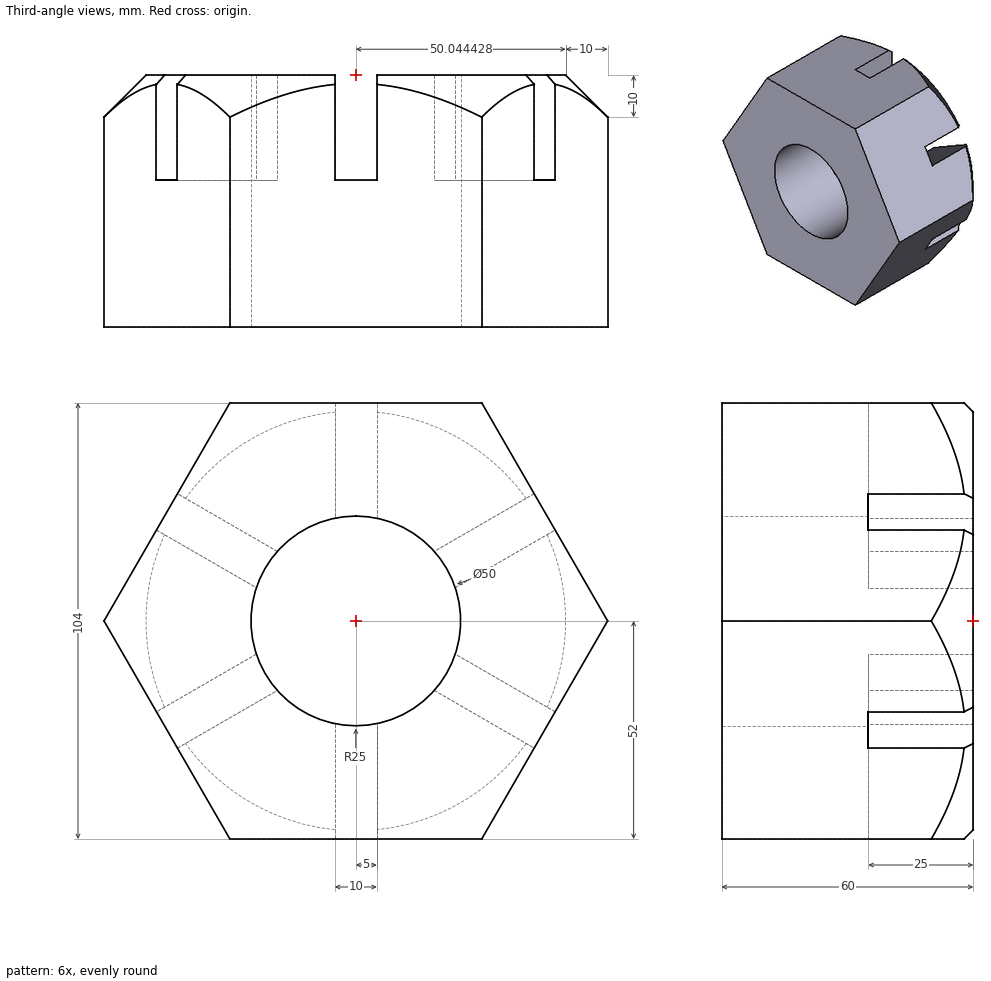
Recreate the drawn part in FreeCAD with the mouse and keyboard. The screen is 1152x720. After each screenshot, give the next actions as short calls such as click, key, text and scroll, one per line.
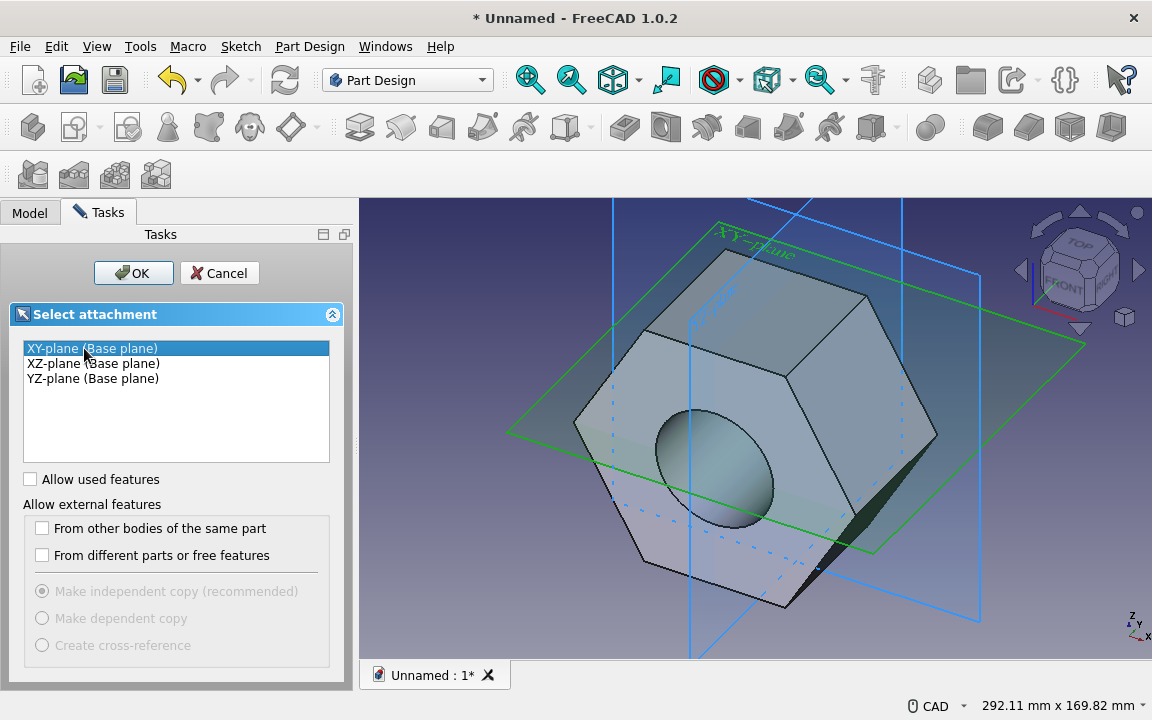
click(134, 273)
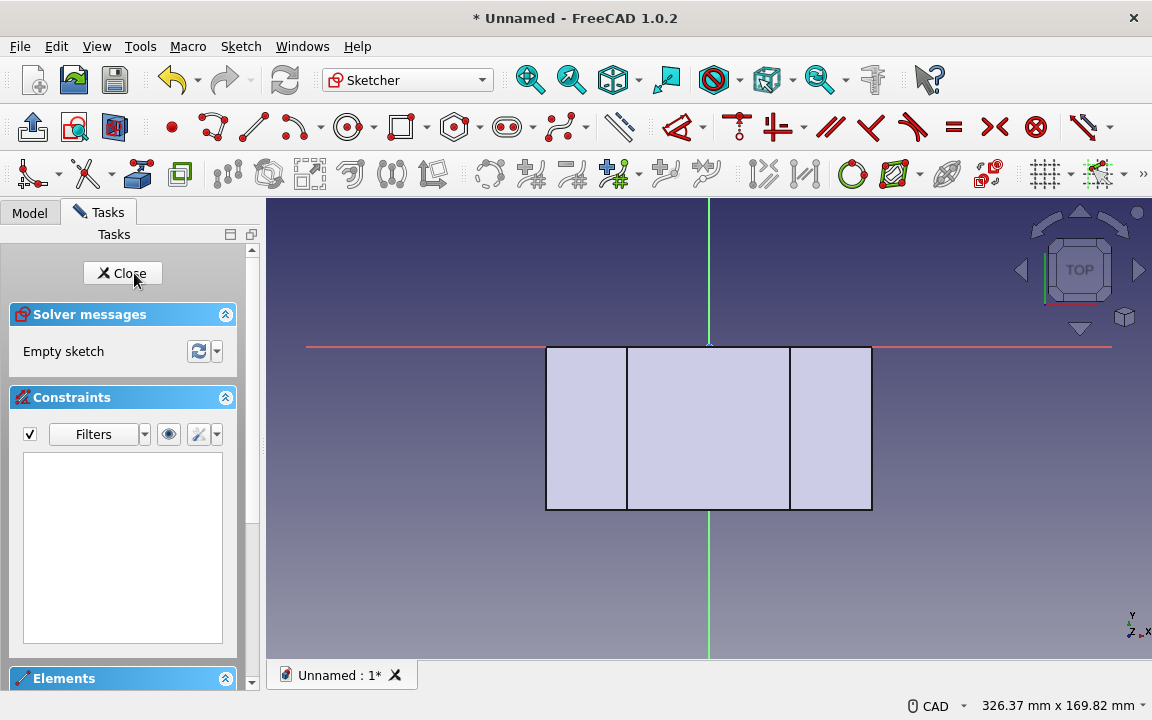
click(115, 128)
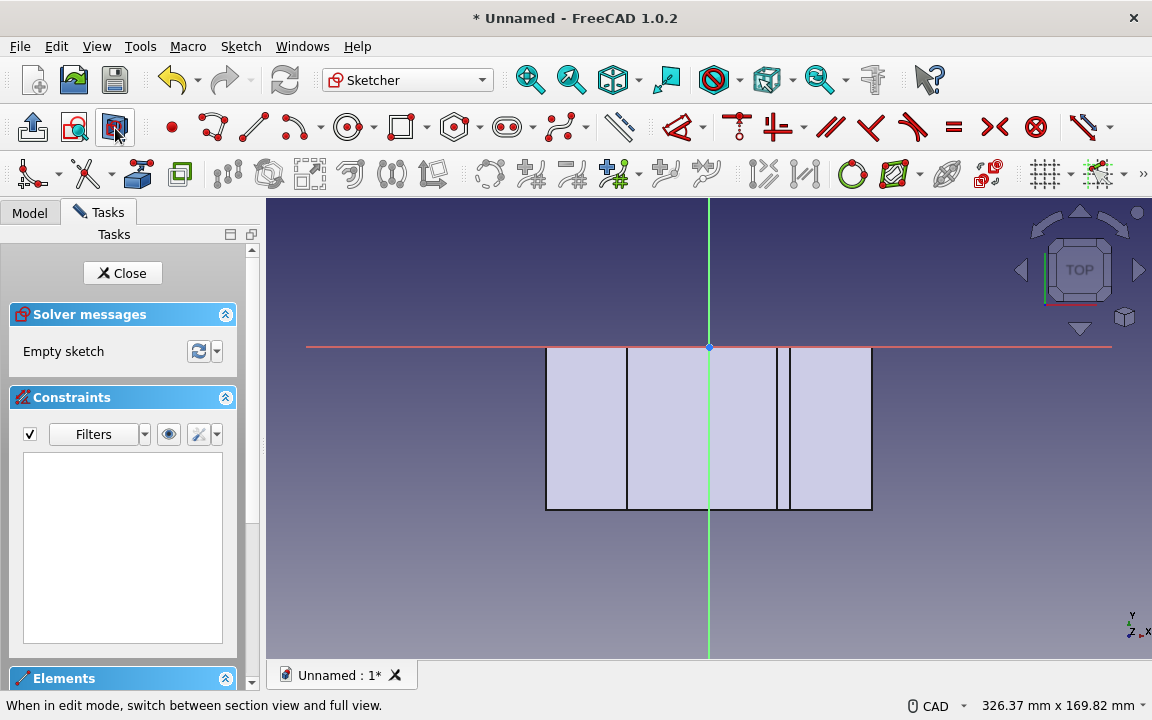
scroll(880, 354, up, 12)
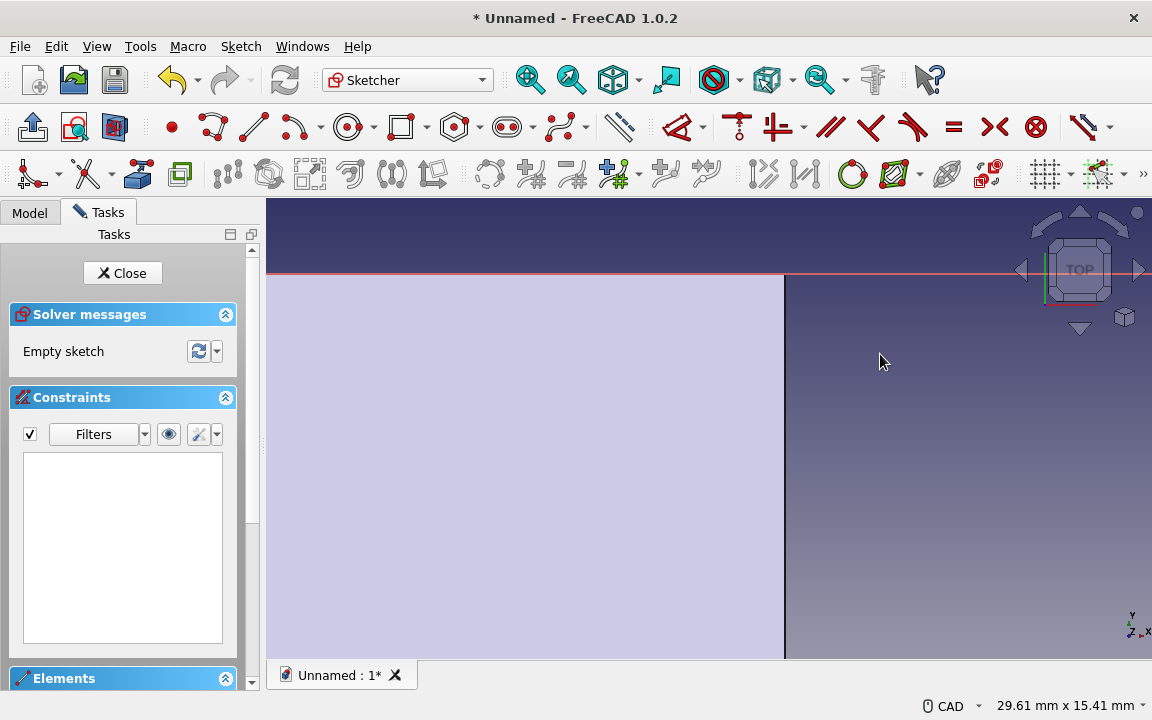
click(213, 128)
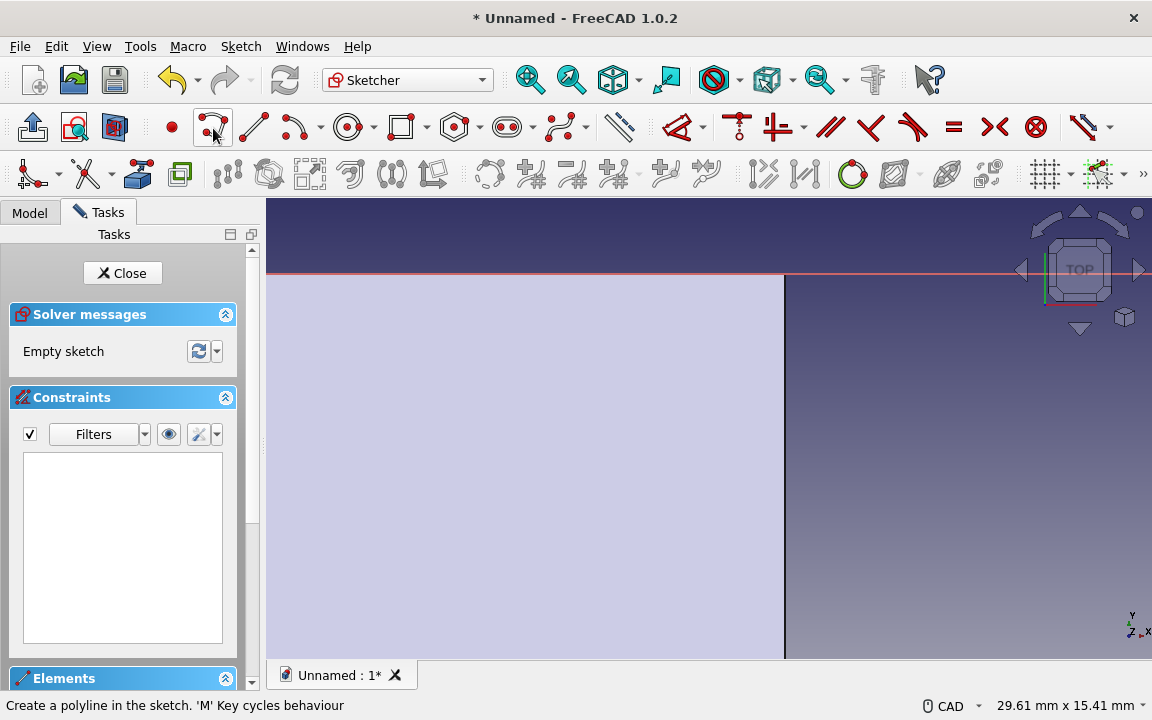
click(486, 274)
click(785, 573)
click(785, 283)
click(486, 274)
key(Escape)
key(Escape)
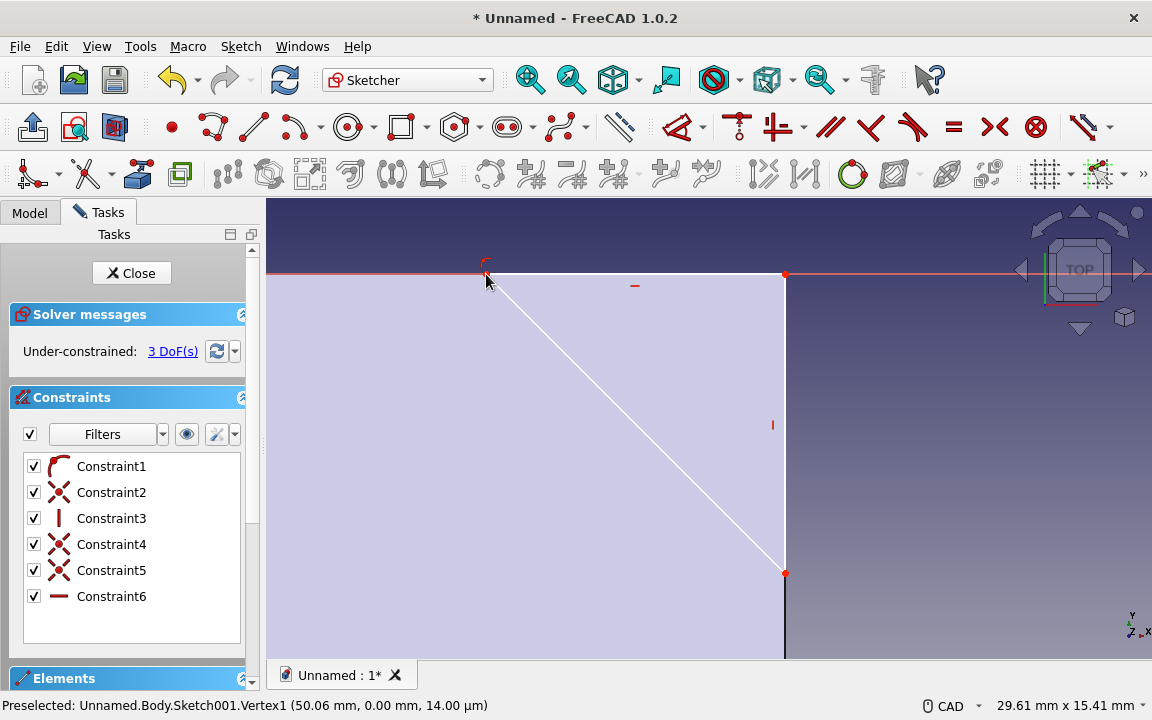
click(676, 128)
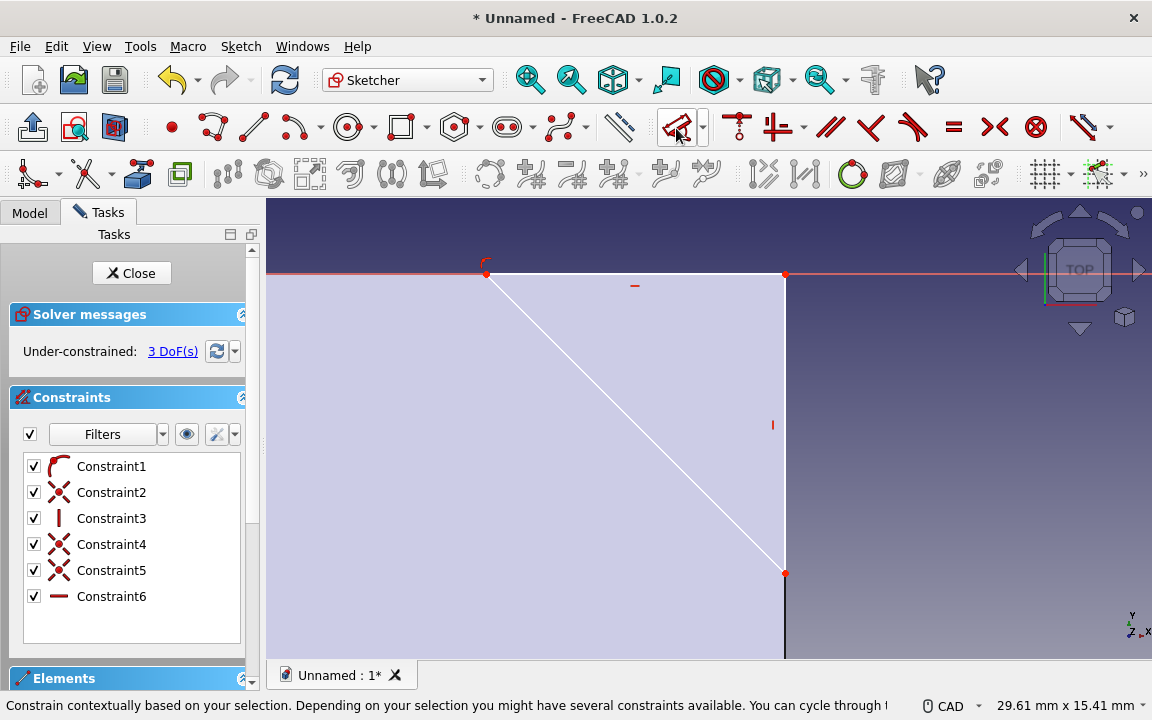
click(785, 484)
click(819, 424)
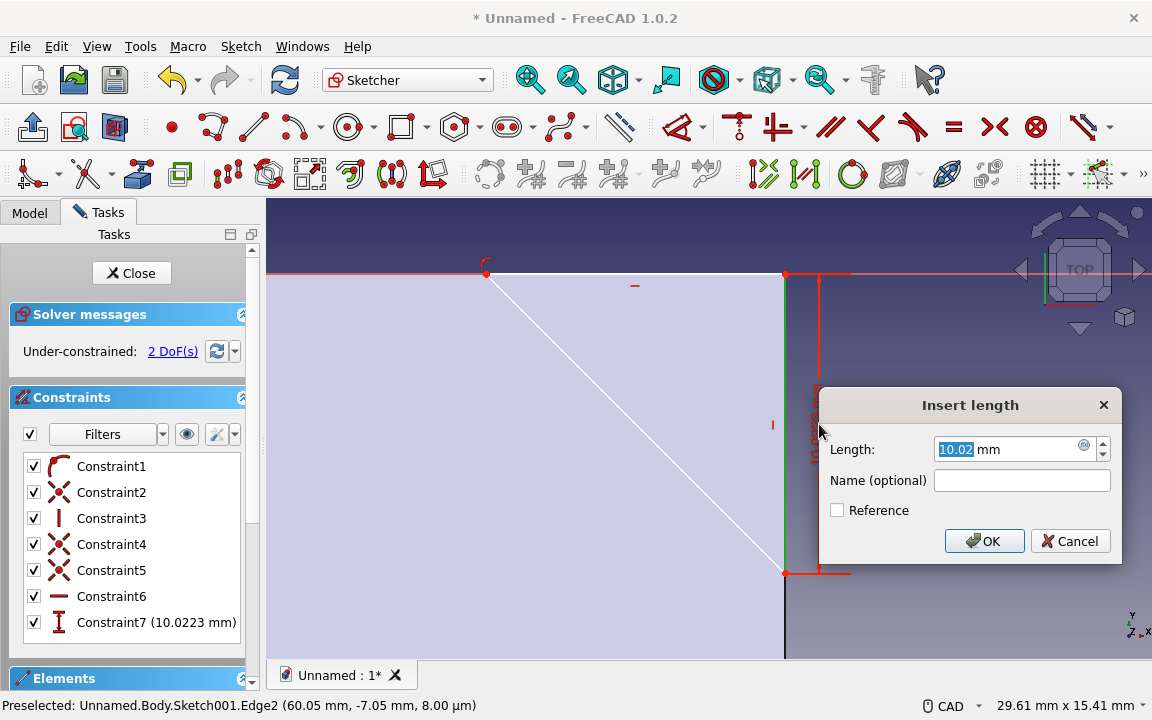
text(10)
key(Return)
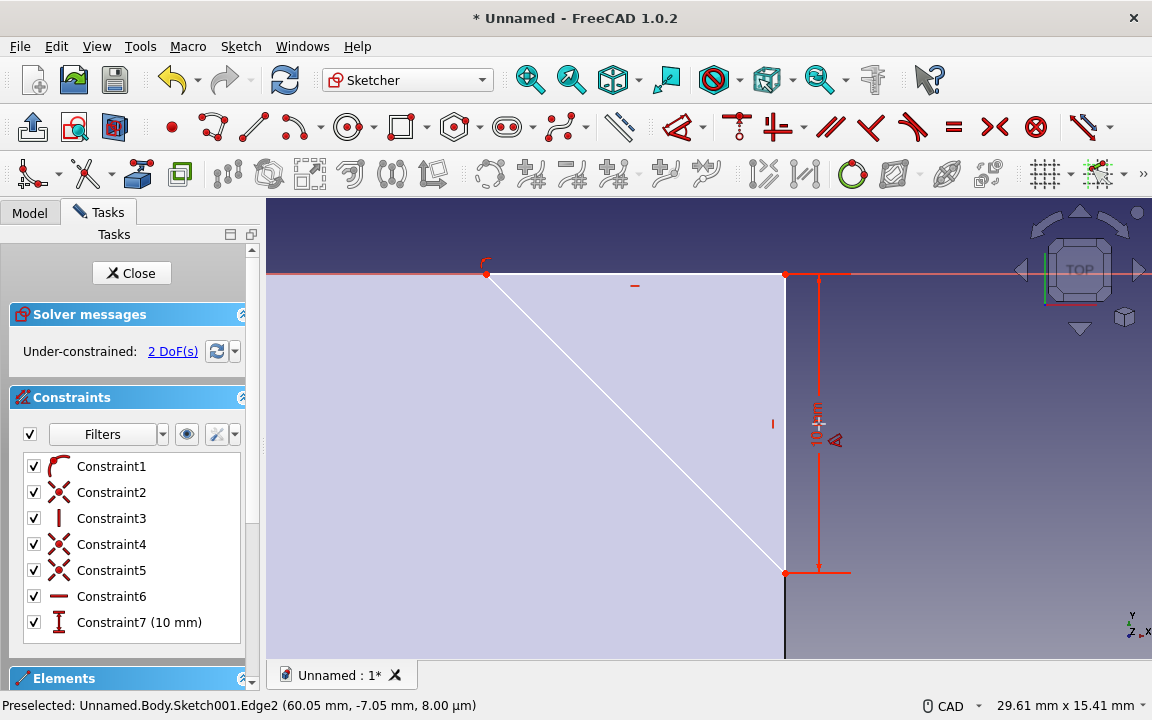
click(695, 274)
click(636, 240)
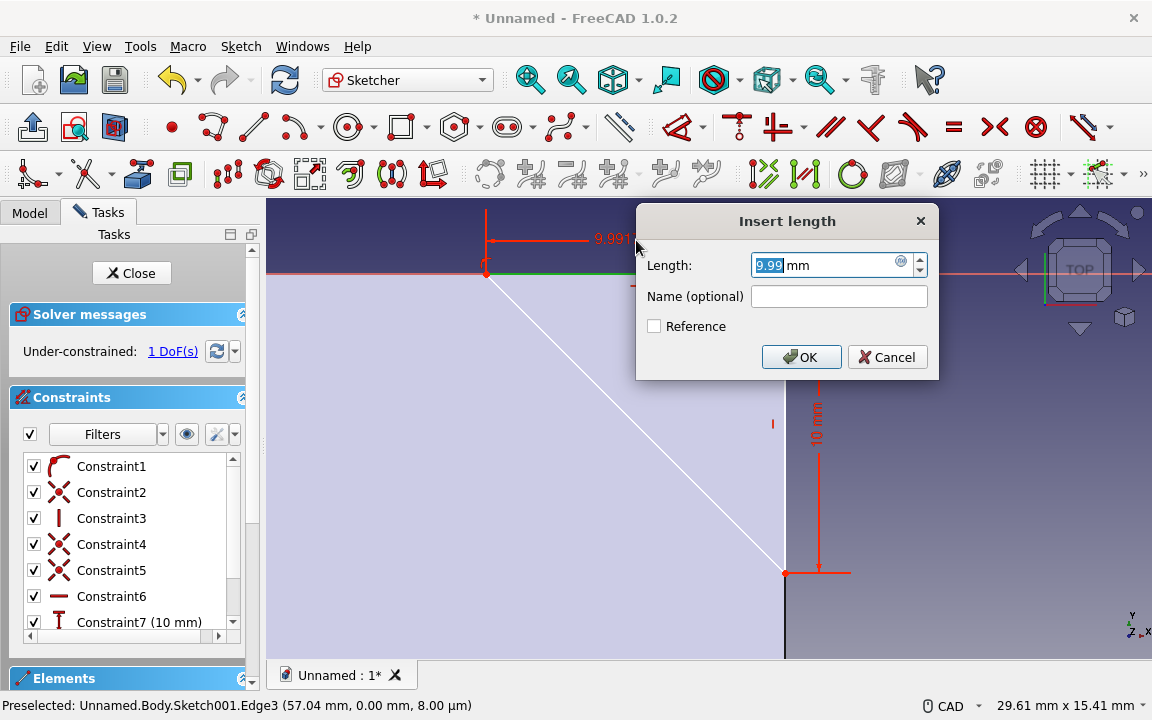
text(10)
key(Return)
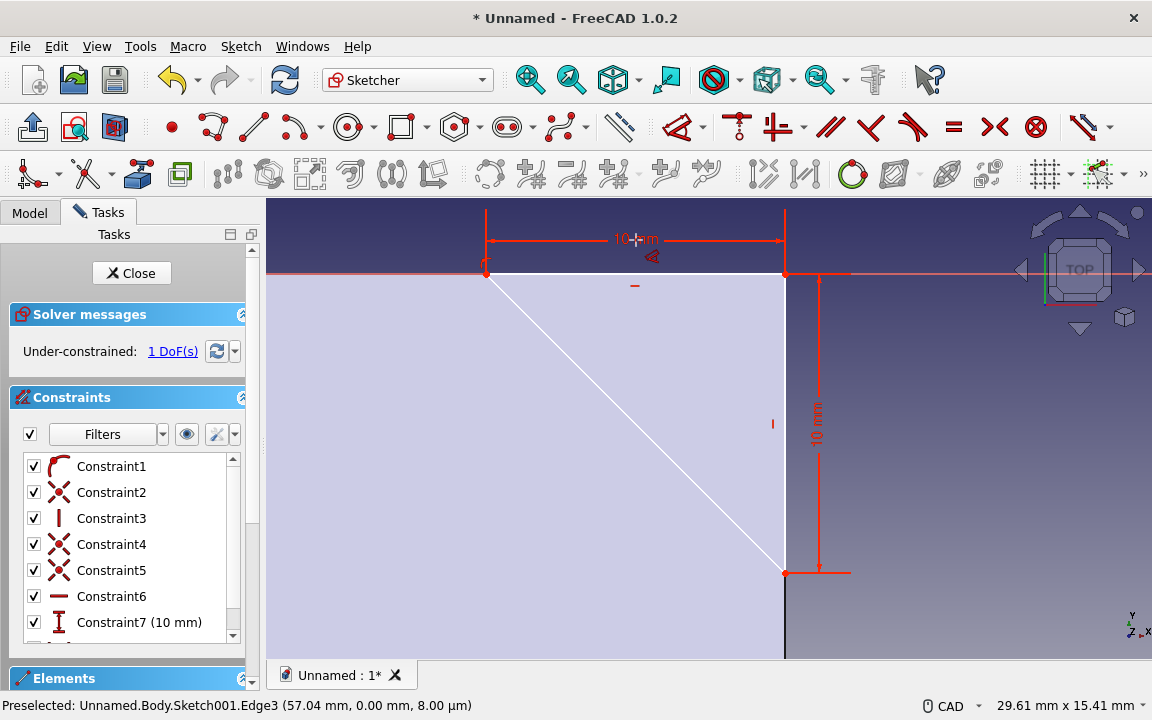
click(486, 274)
click(390, 240)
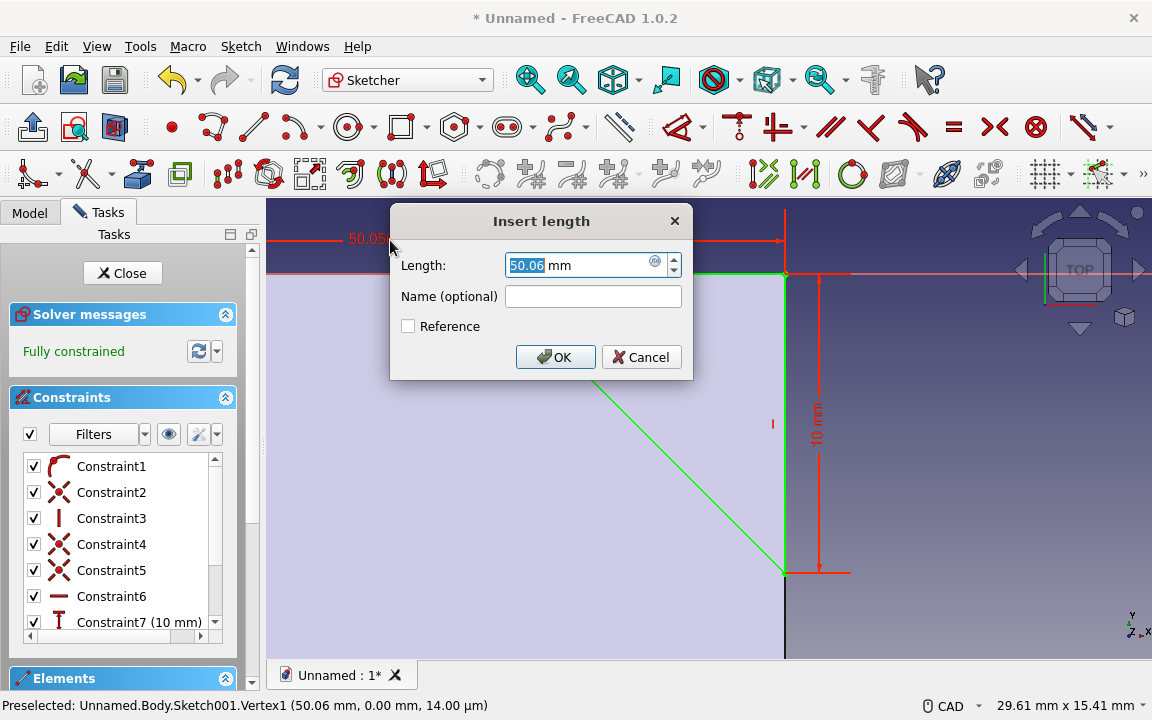
text(50.044428)
key(Return)
key(Escape)